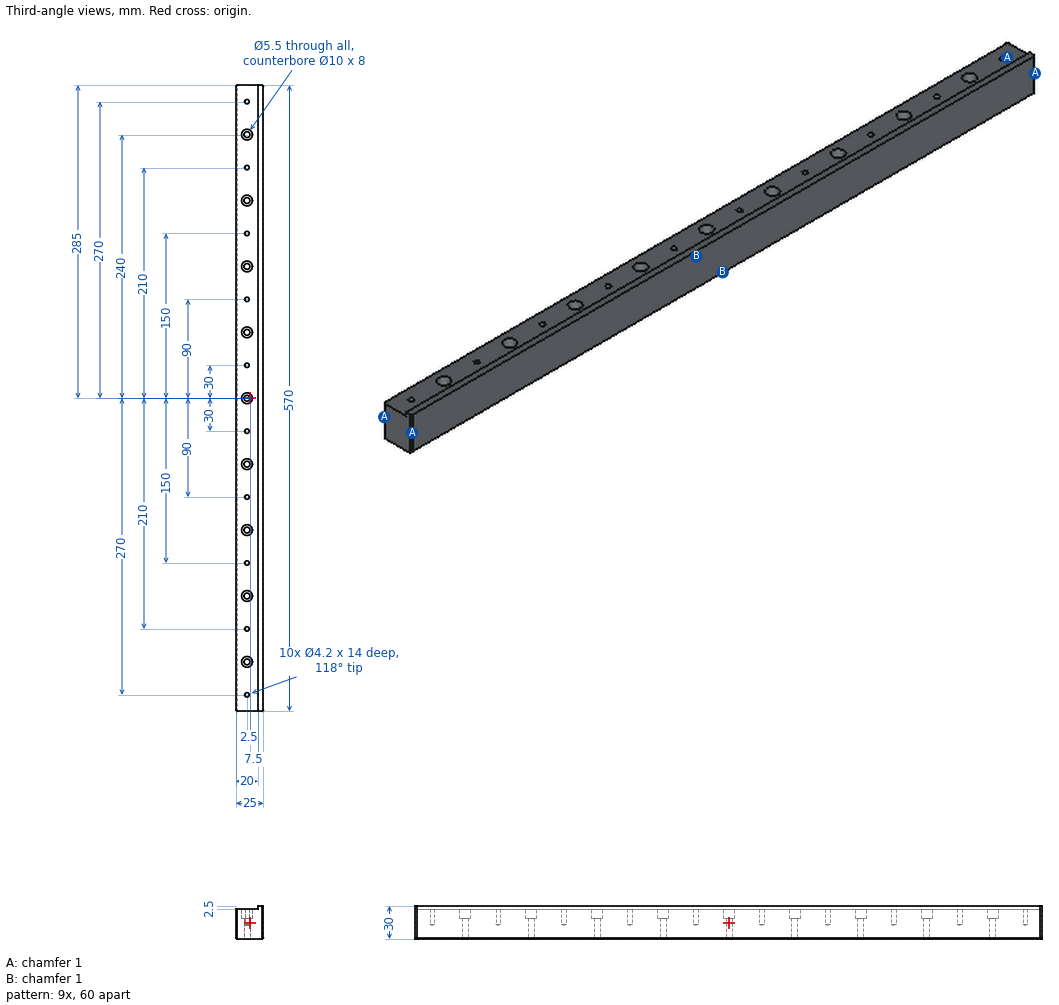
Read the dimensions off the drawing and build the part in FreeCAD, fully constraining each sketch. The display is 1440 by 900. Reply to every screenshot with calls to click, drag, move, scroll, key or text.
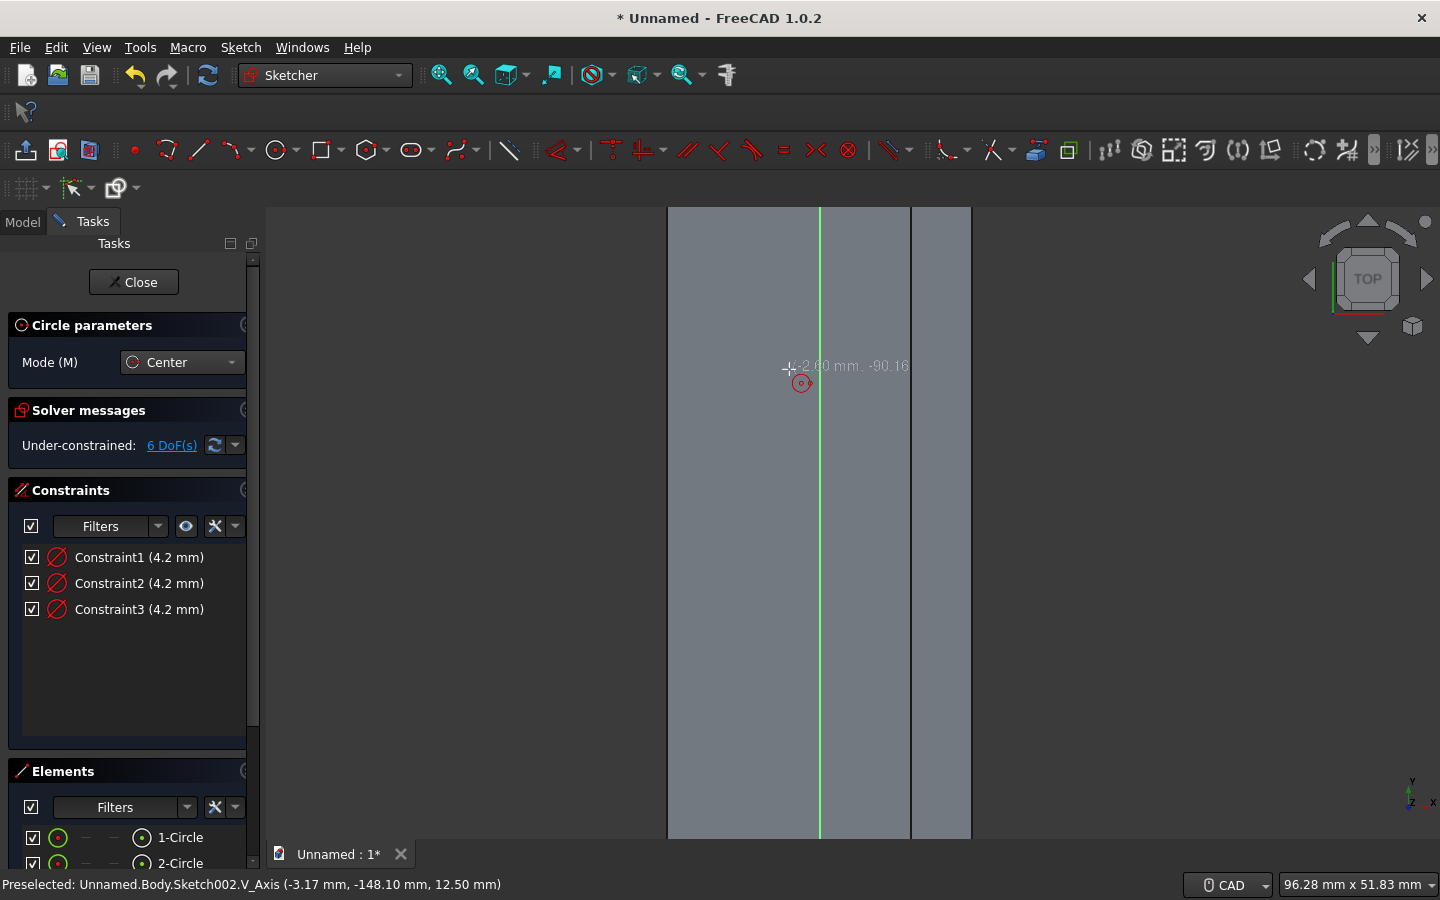
click(789, 369)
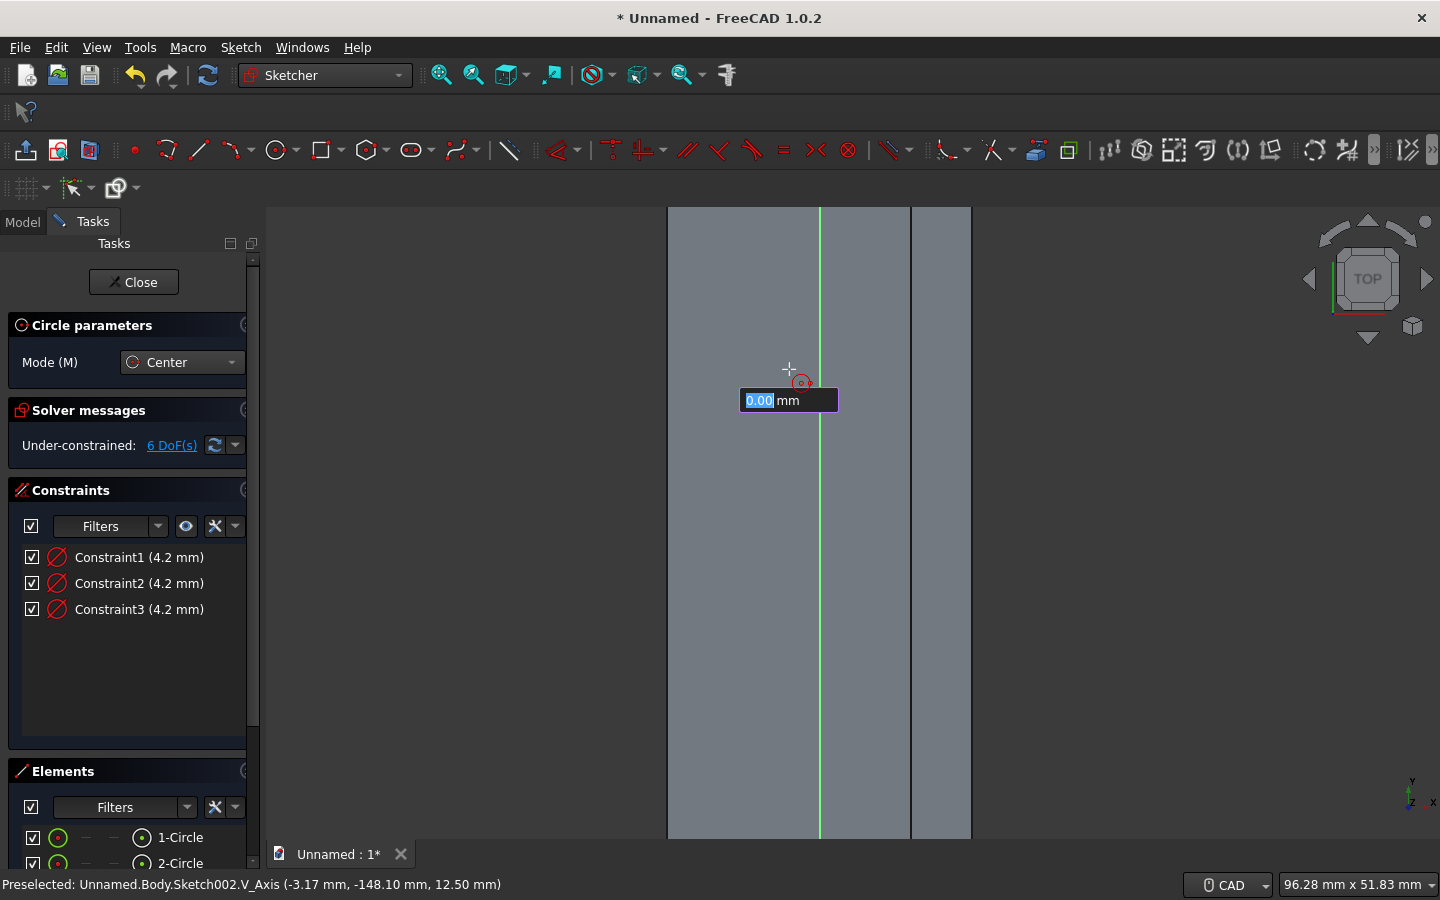
scroll(784, 604, down, 14)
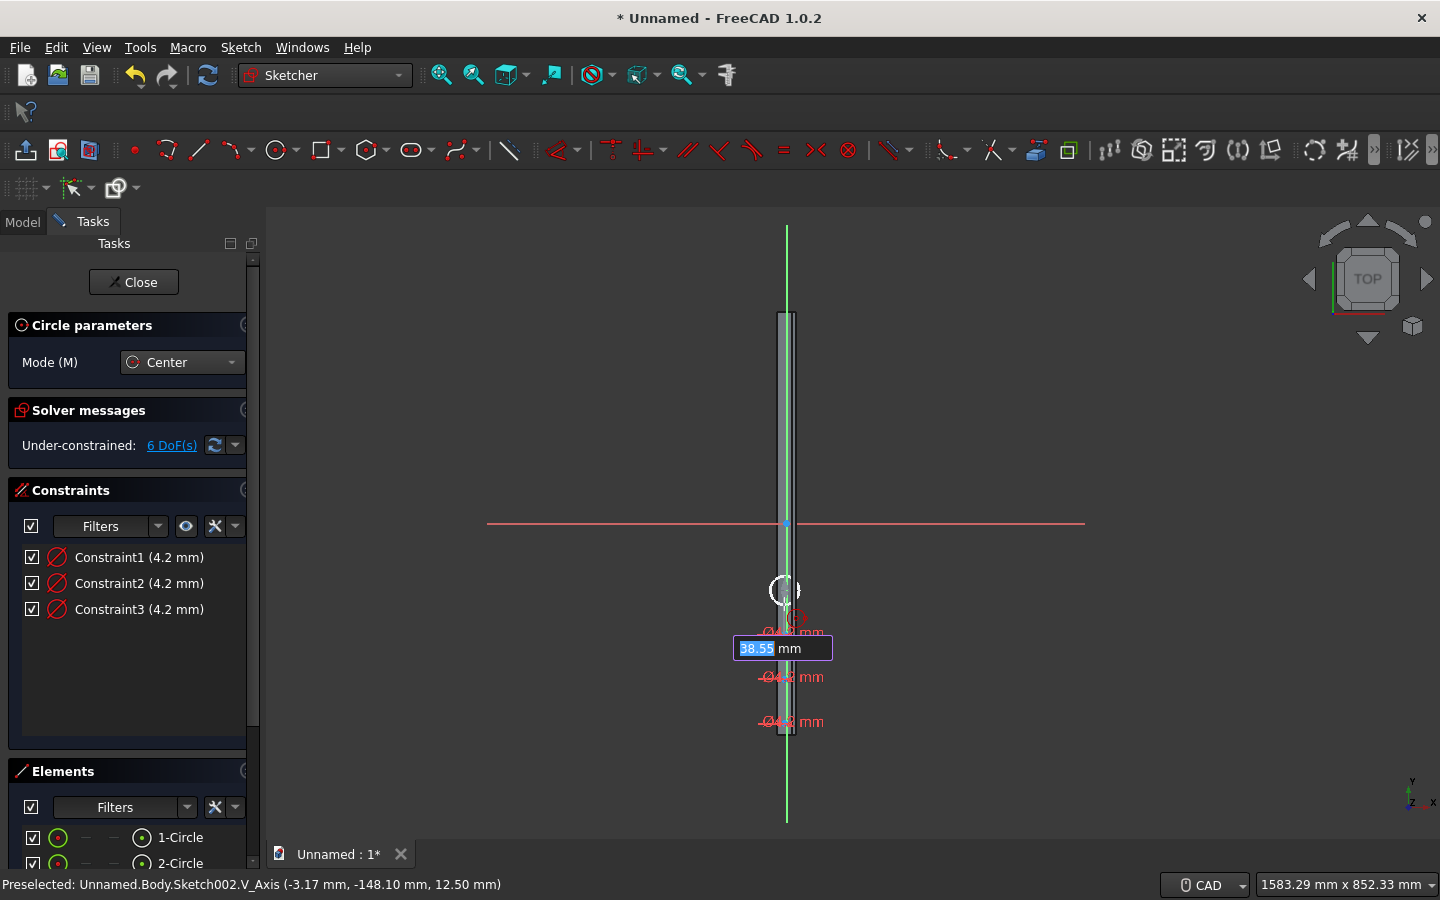
scroll(784, 589, up, 9)
move(780, 587)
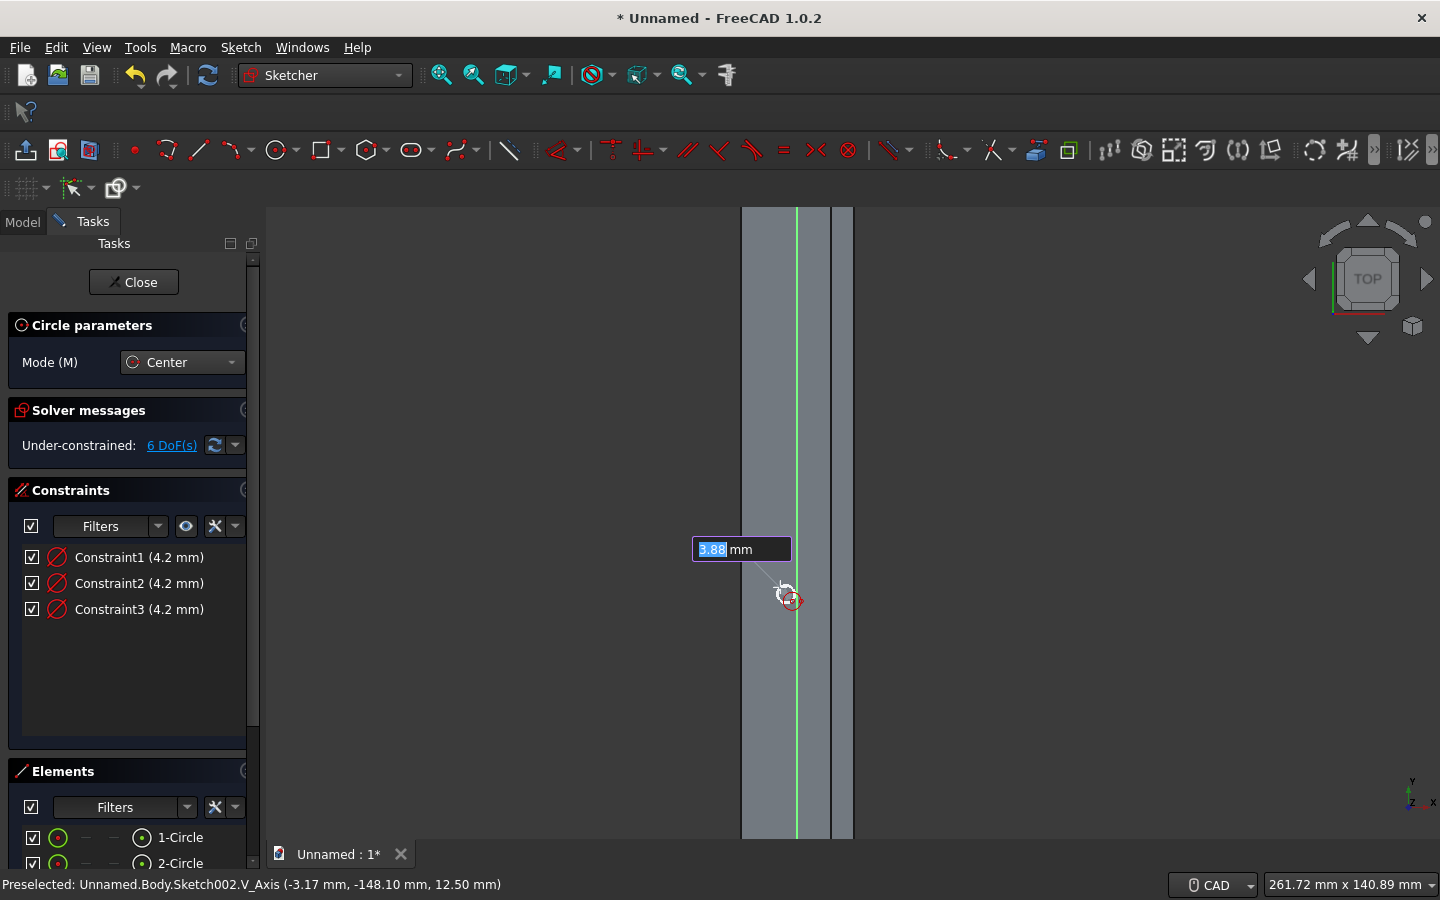
text(4.2)
key(Return)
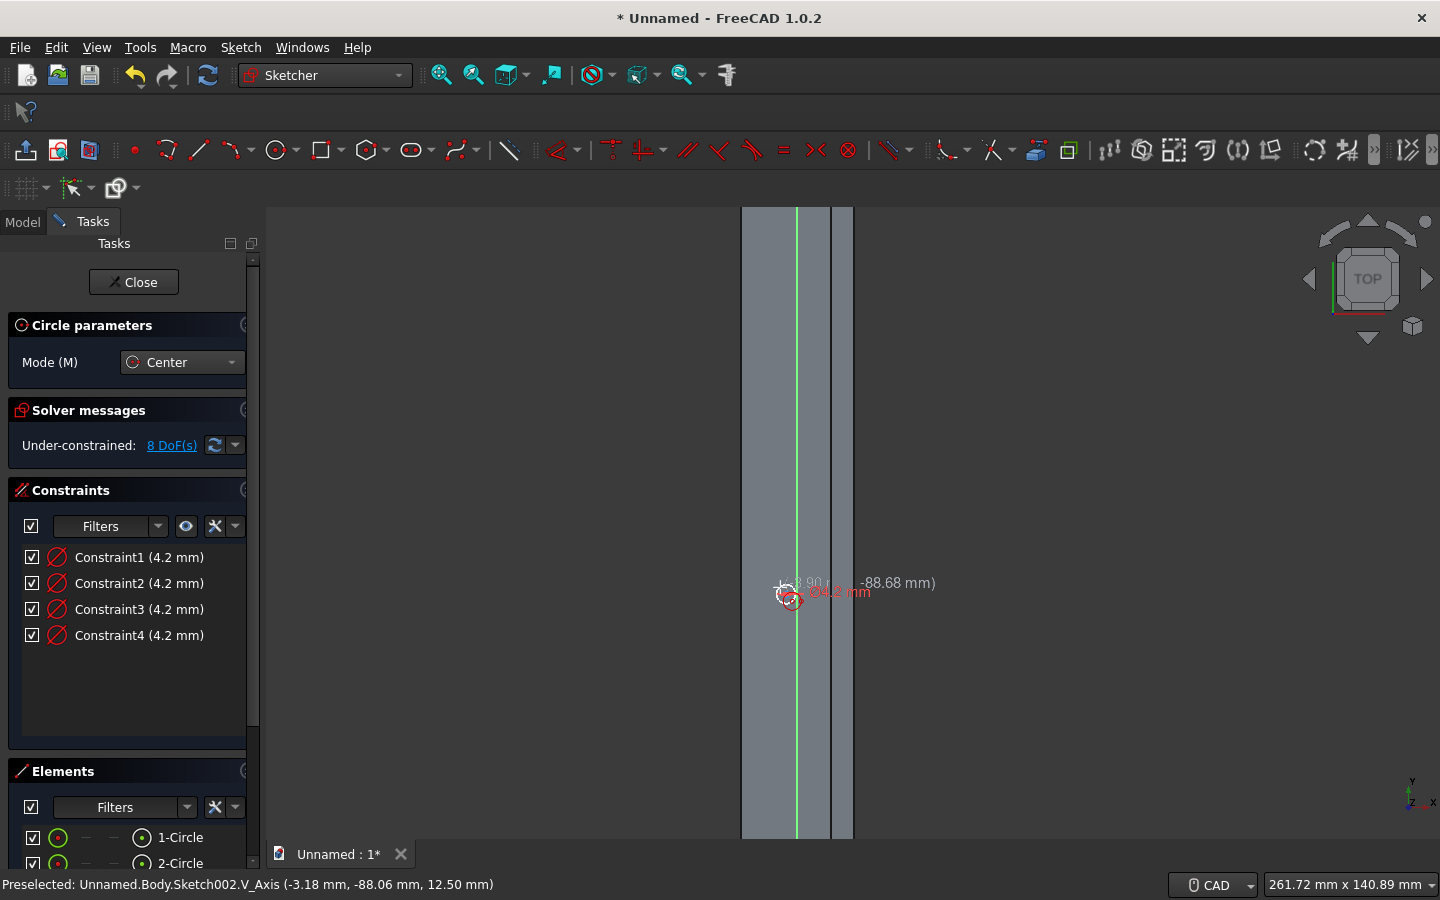
scroll(786, 325, up, 5)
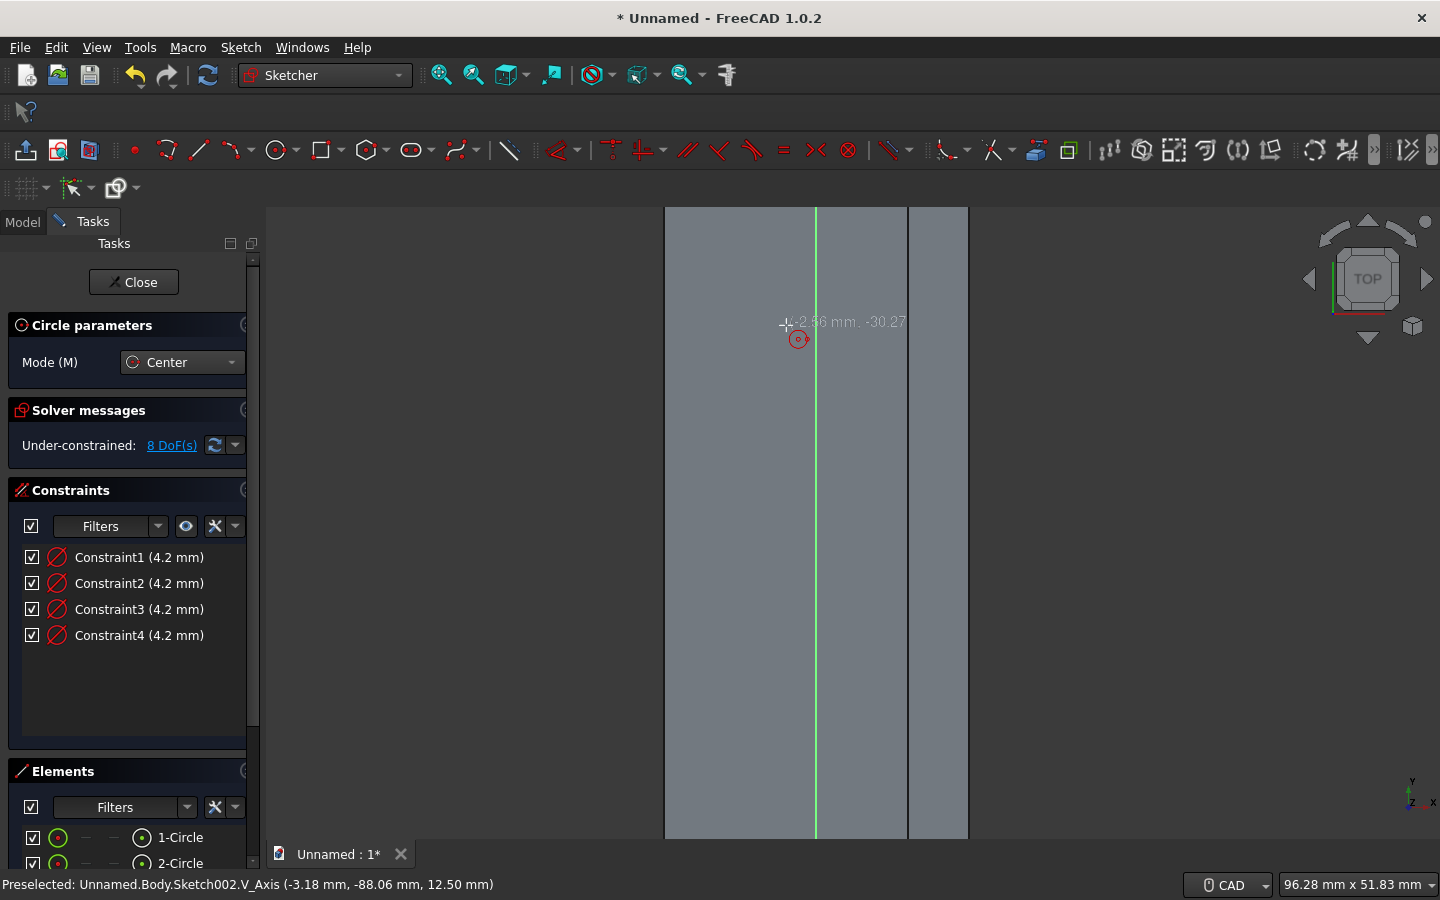
click(786, 324)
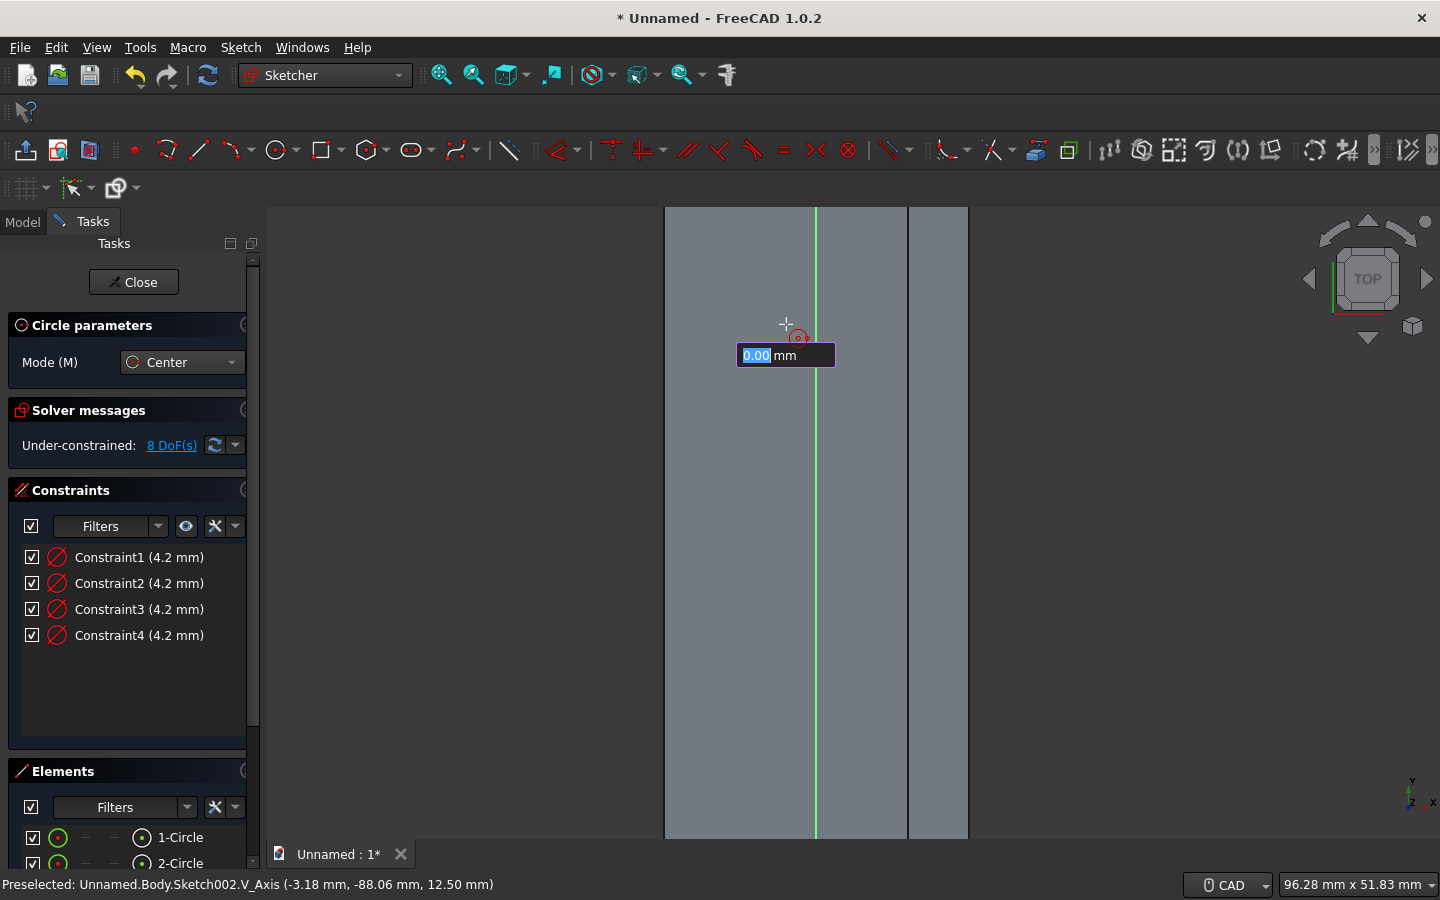
scroll(784, 560, down, 14)